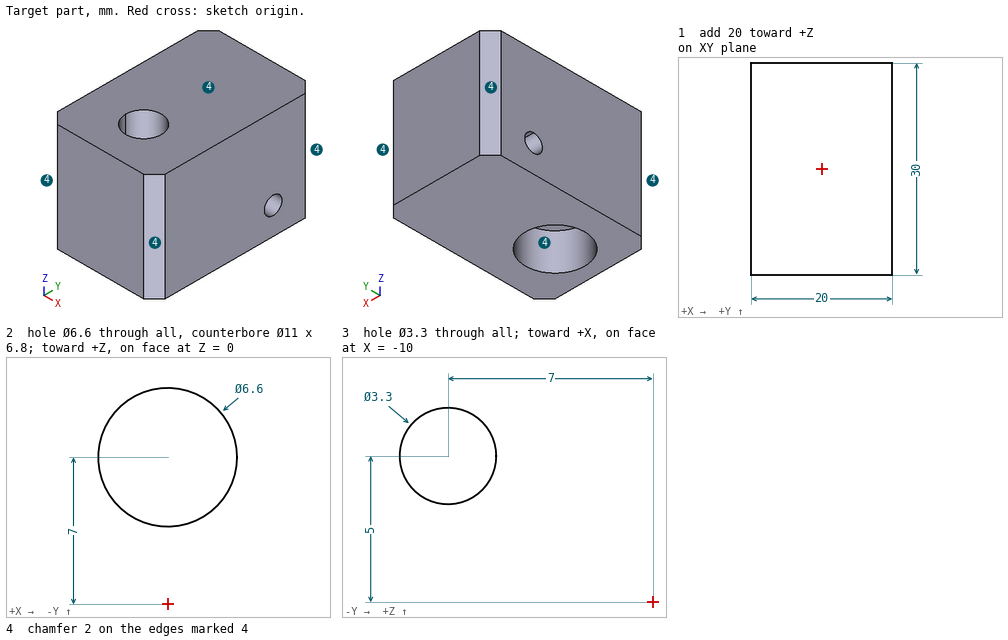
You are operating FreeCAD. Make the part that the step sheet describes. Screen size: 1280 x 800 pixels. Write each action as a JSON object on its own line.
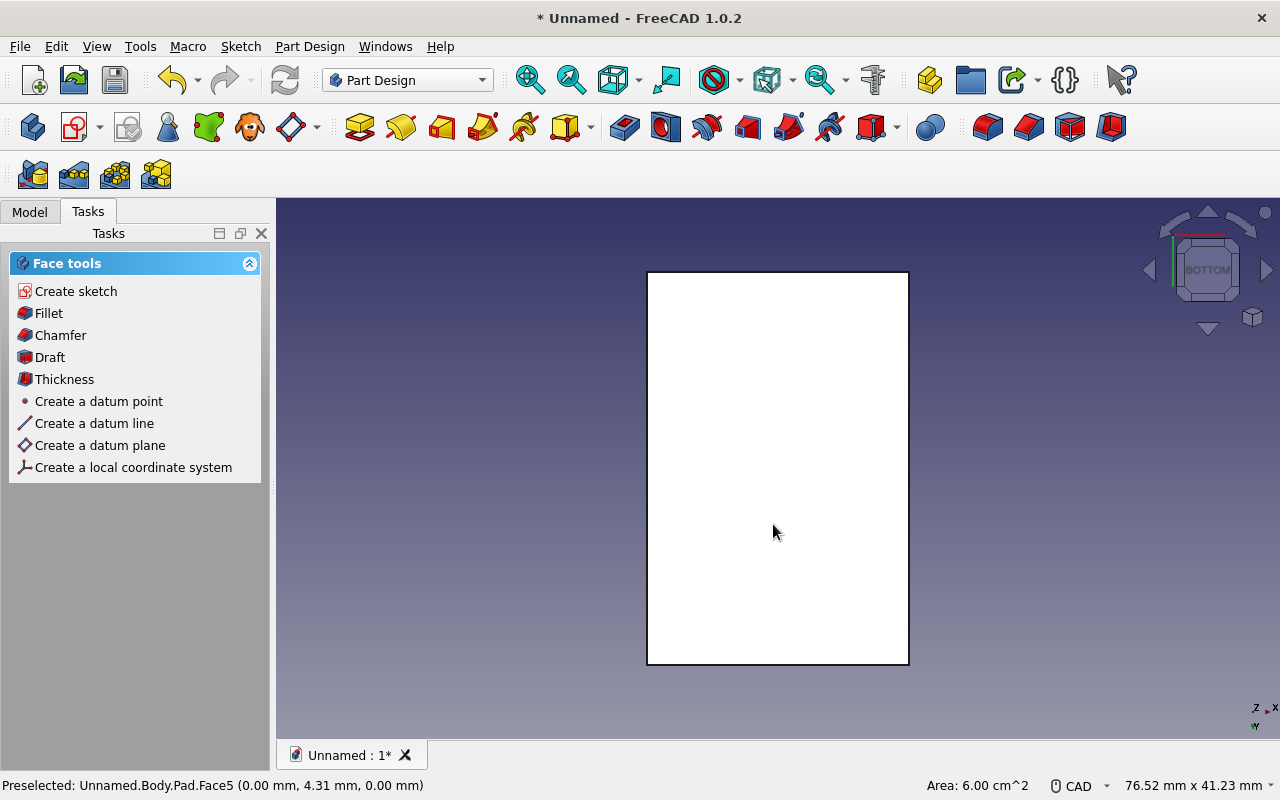
{"action": "left_click", "coordinate": [74, 128]}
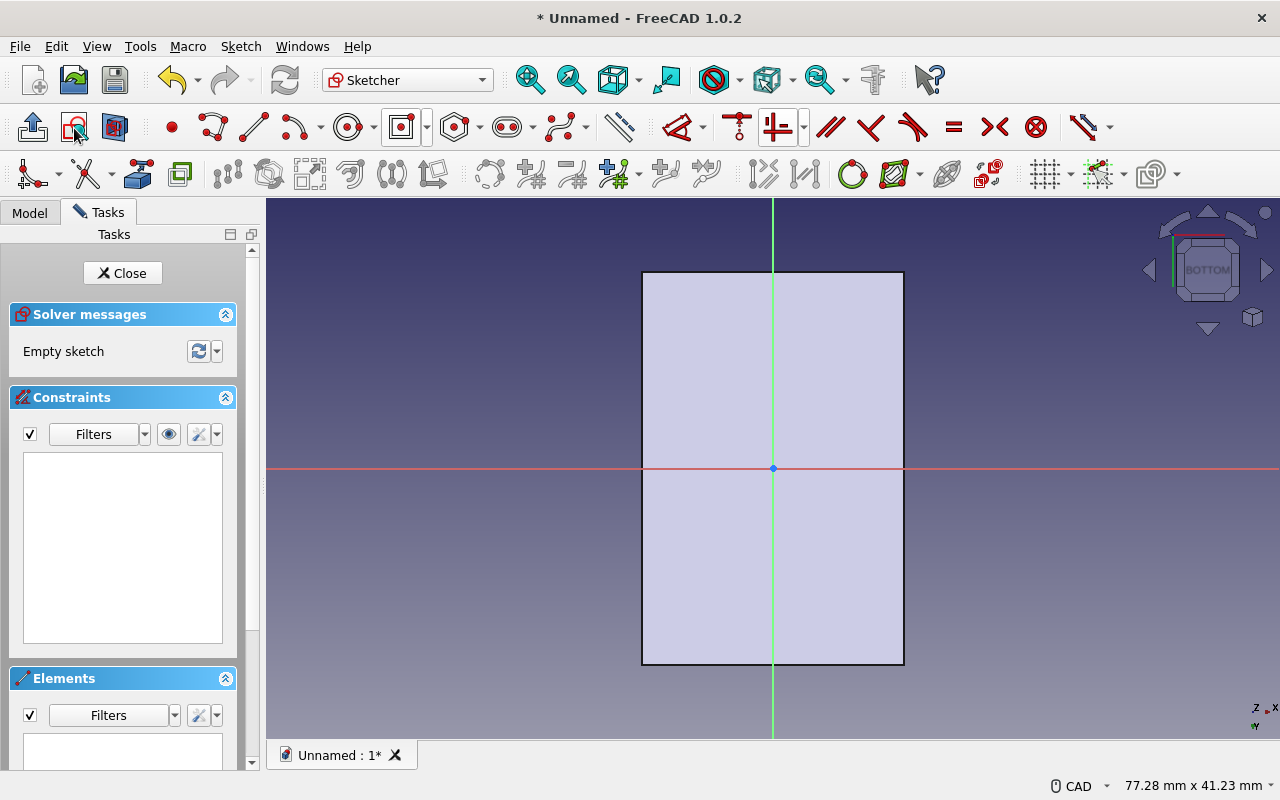
{"action": "scroll", "coordinate": [813, 362], "scroll_direction": "up", "scroll_amount": 5}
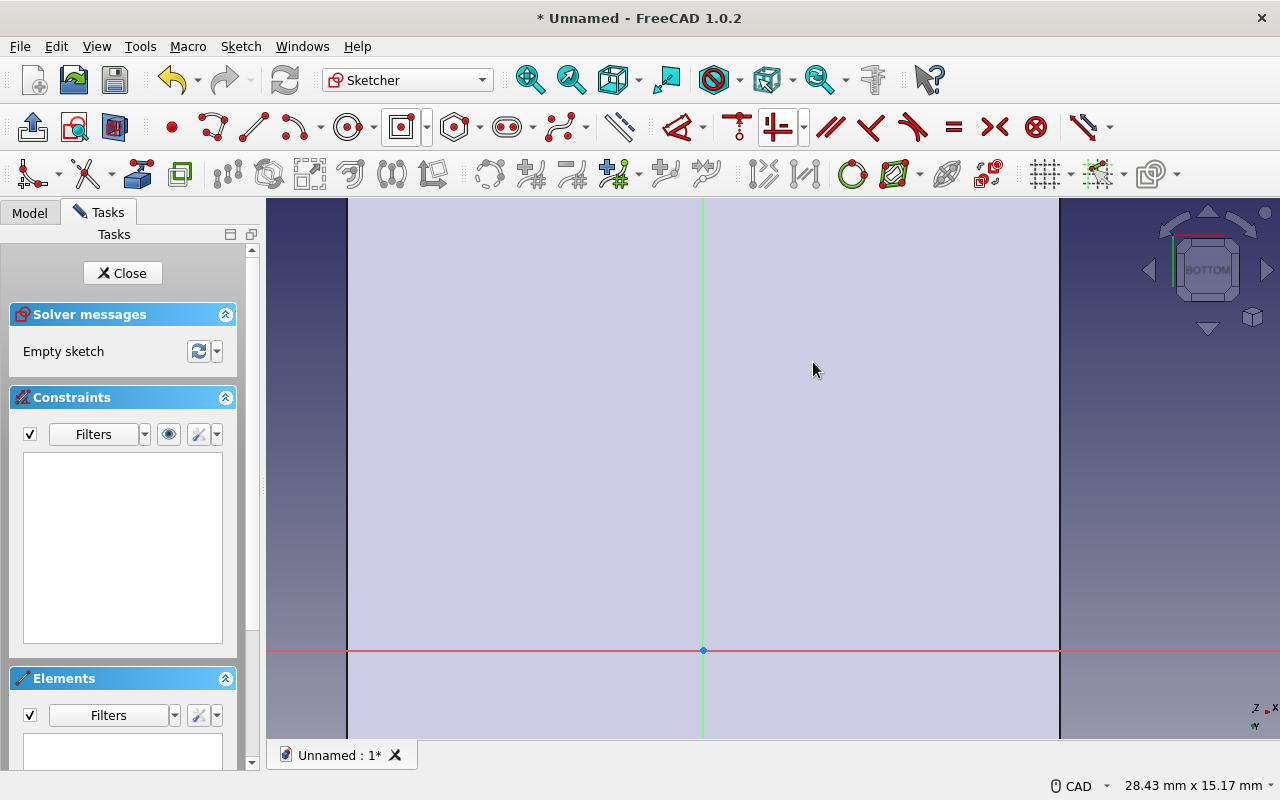
{"action": "key", "text": "g c"}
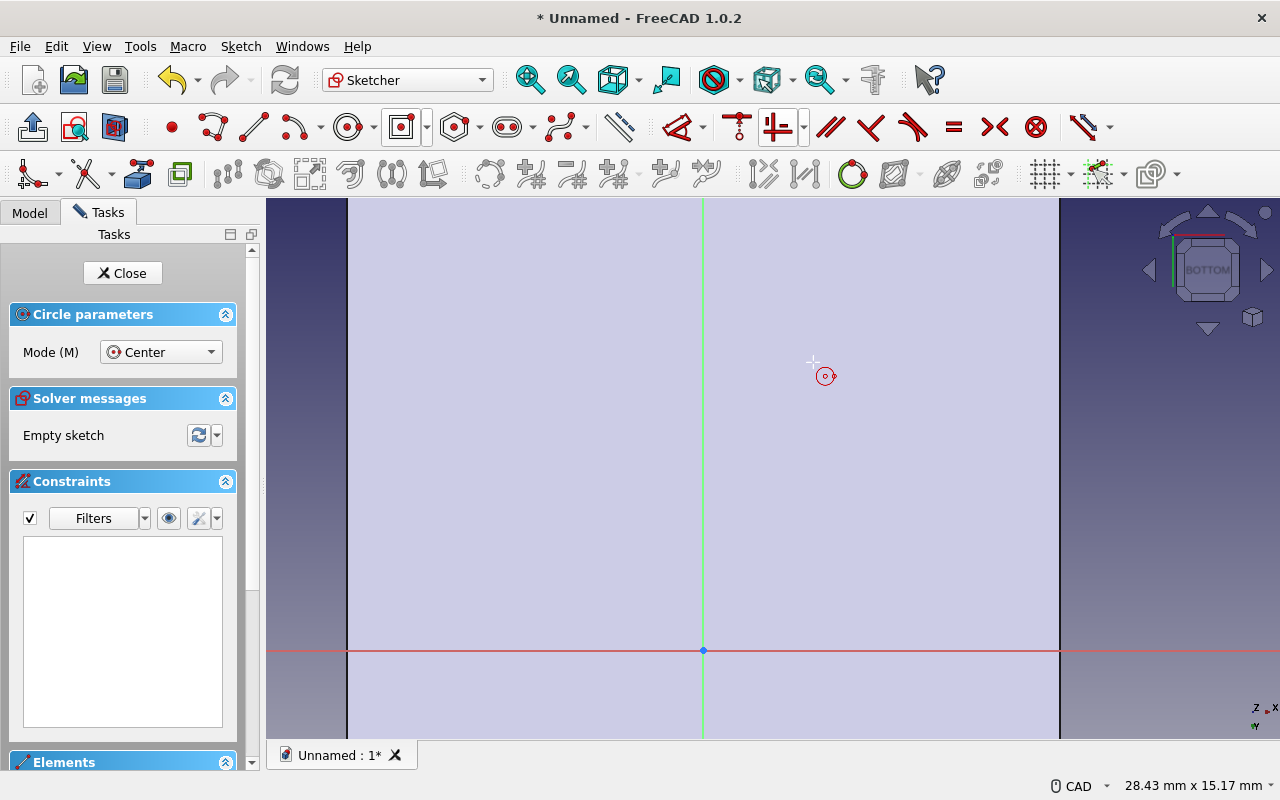
{"action": "left_click", "coordinate": [703, 401]}
{"action": "left_click", "coordinate": [787, 318]}
{"action": "key", "text": "Escape"}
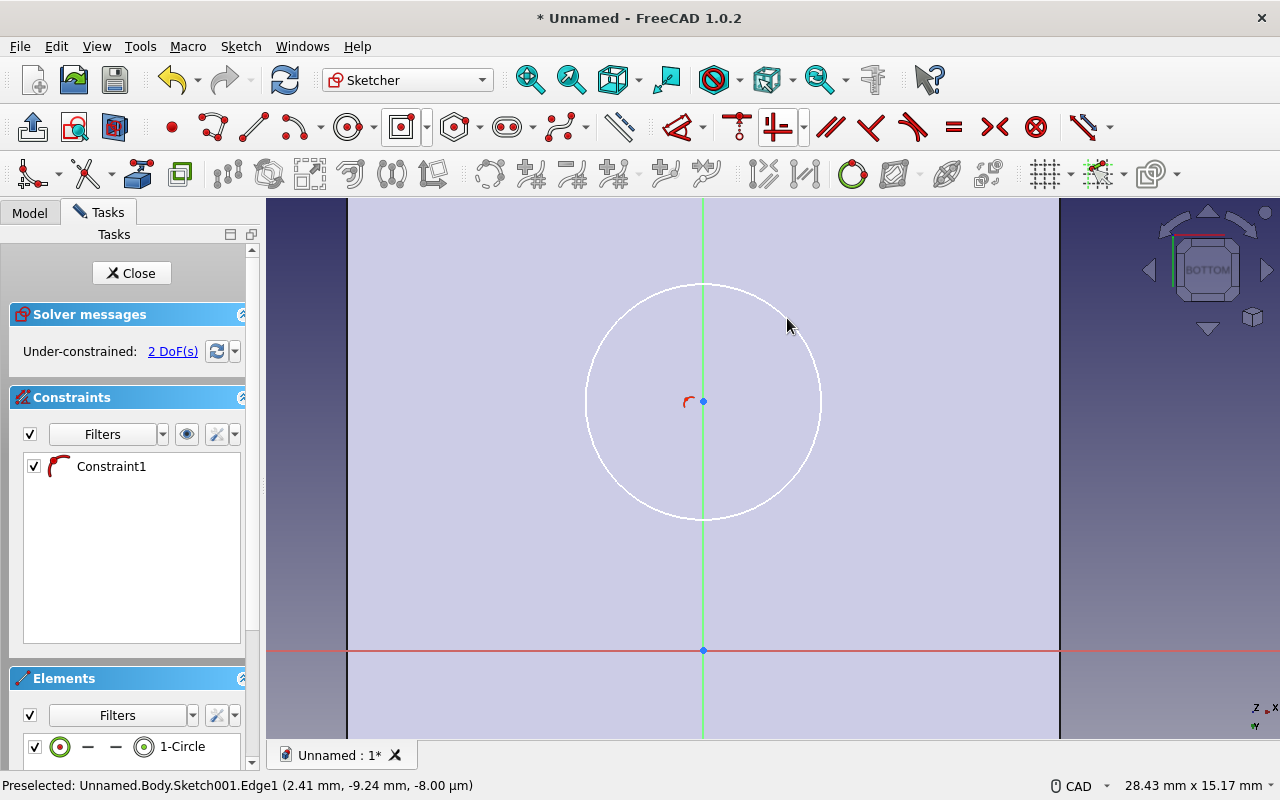
{"action": "left_click", "coordinate": [786, 318]}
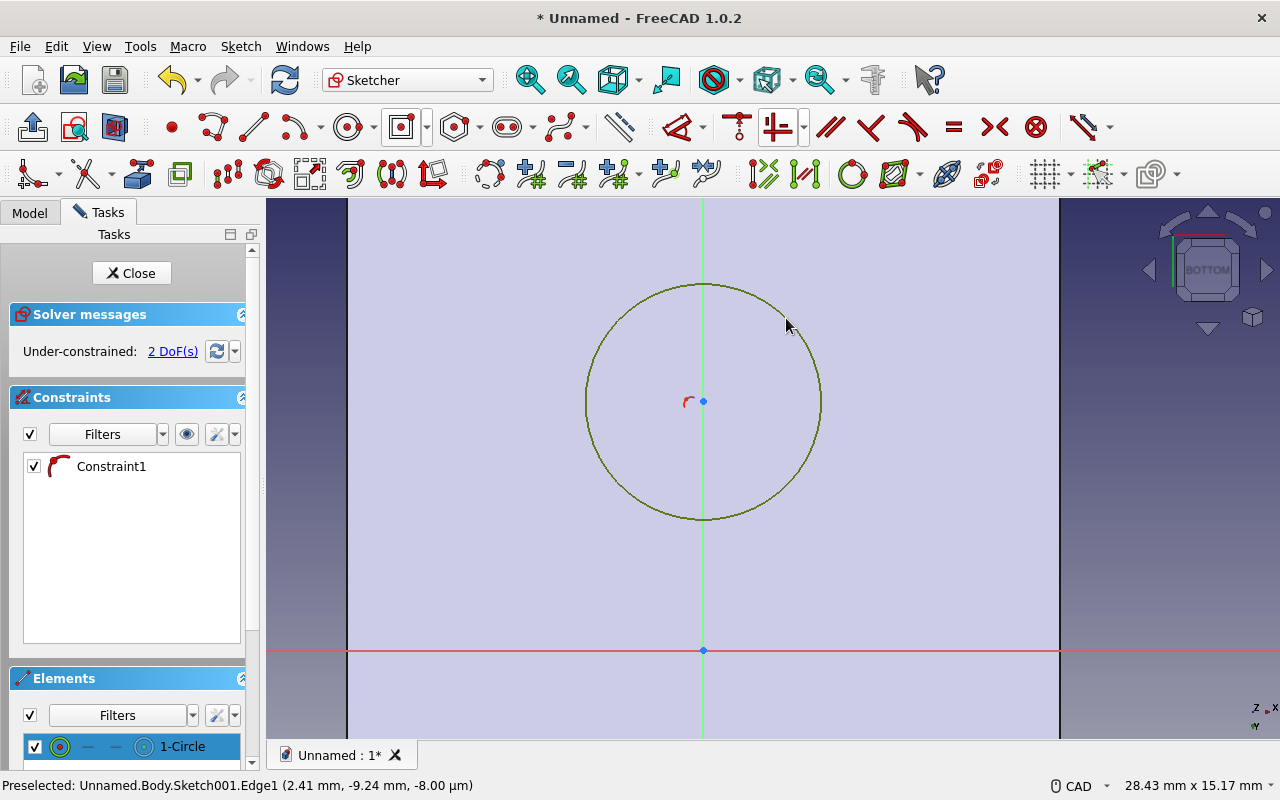
{"action": "left_click", "coordinate": [702, 128]}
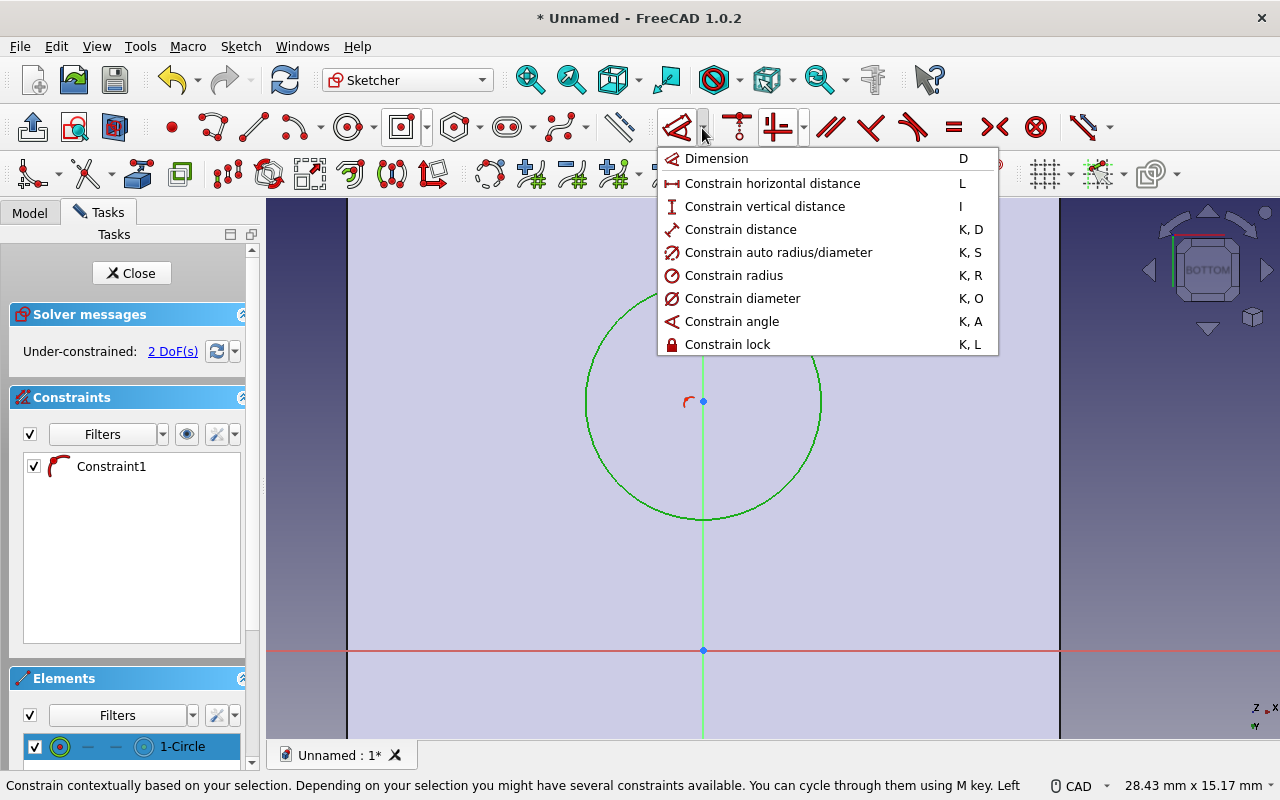
{"action": "left_click", "coordinate": [828, 298]}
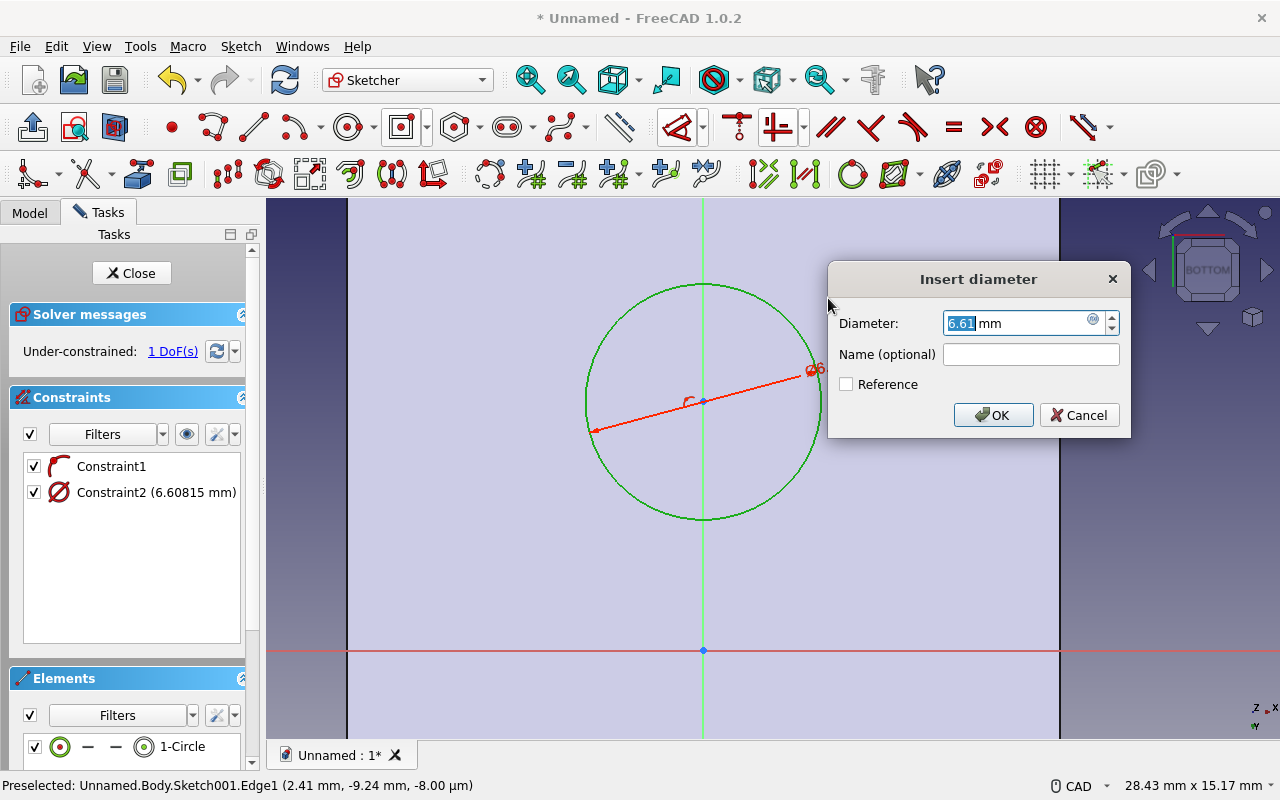
{"action": "type", "text": "6.6"}
{"action": "key", "text": "Return"}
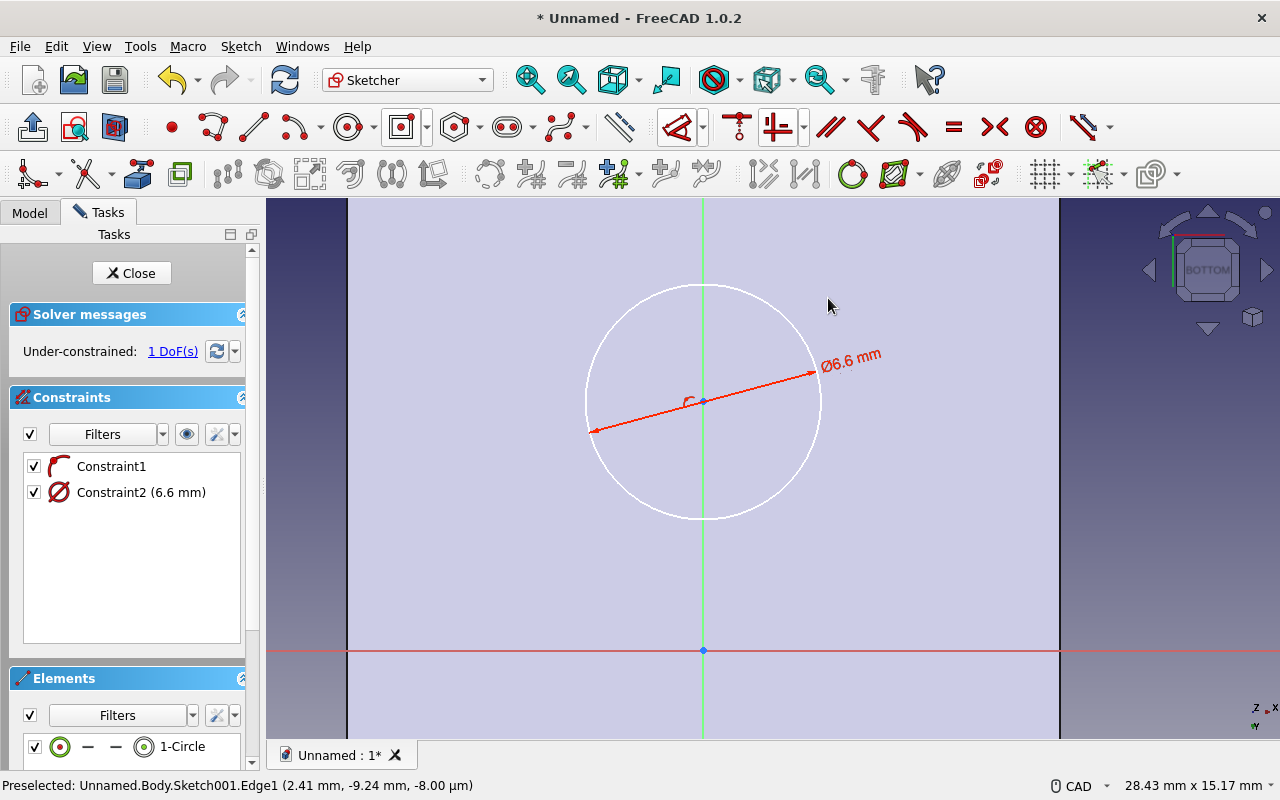
{"action": "left_click", "coordinate": [703, 402]}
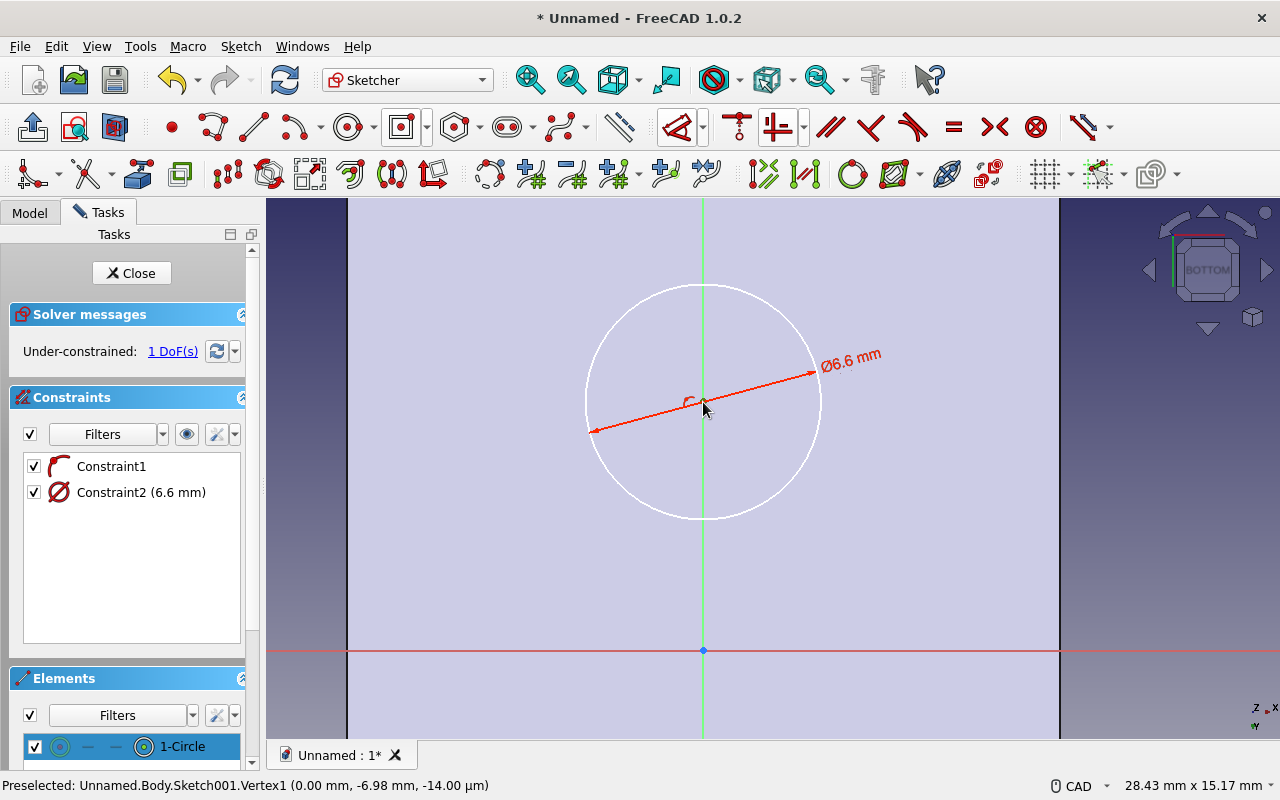
{"action": "key", "text": "i"}